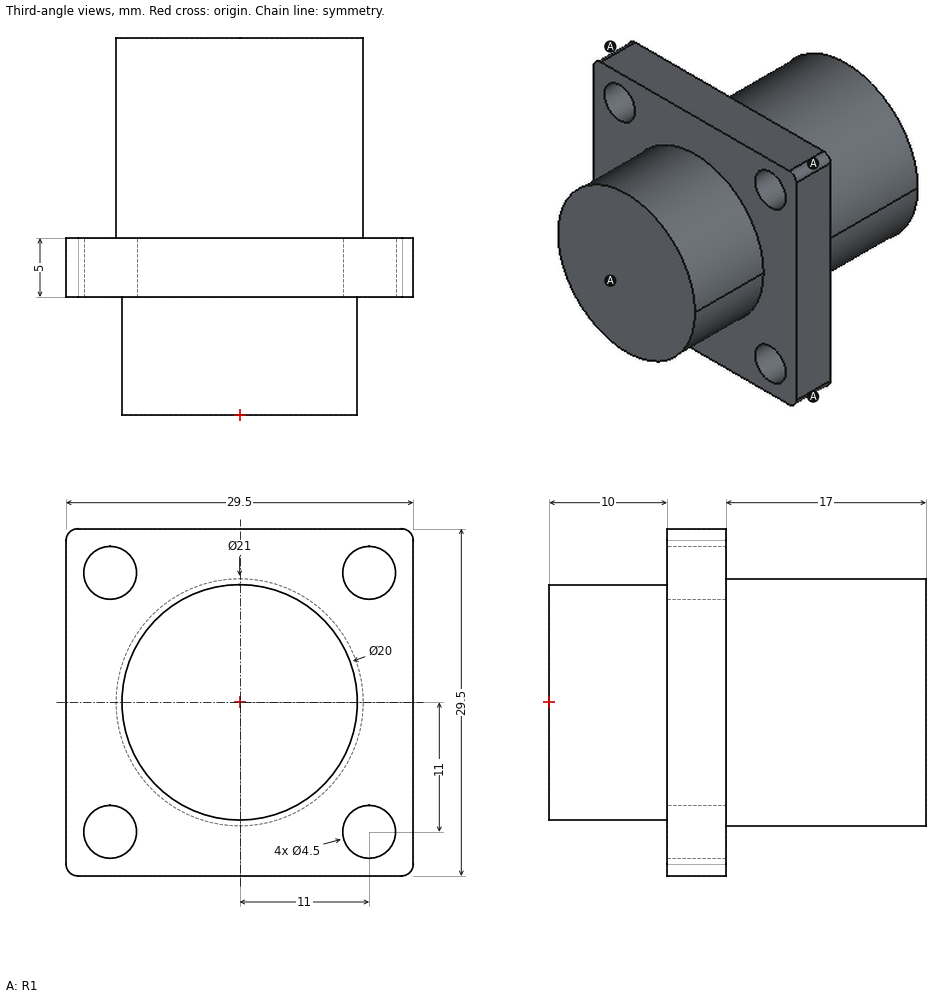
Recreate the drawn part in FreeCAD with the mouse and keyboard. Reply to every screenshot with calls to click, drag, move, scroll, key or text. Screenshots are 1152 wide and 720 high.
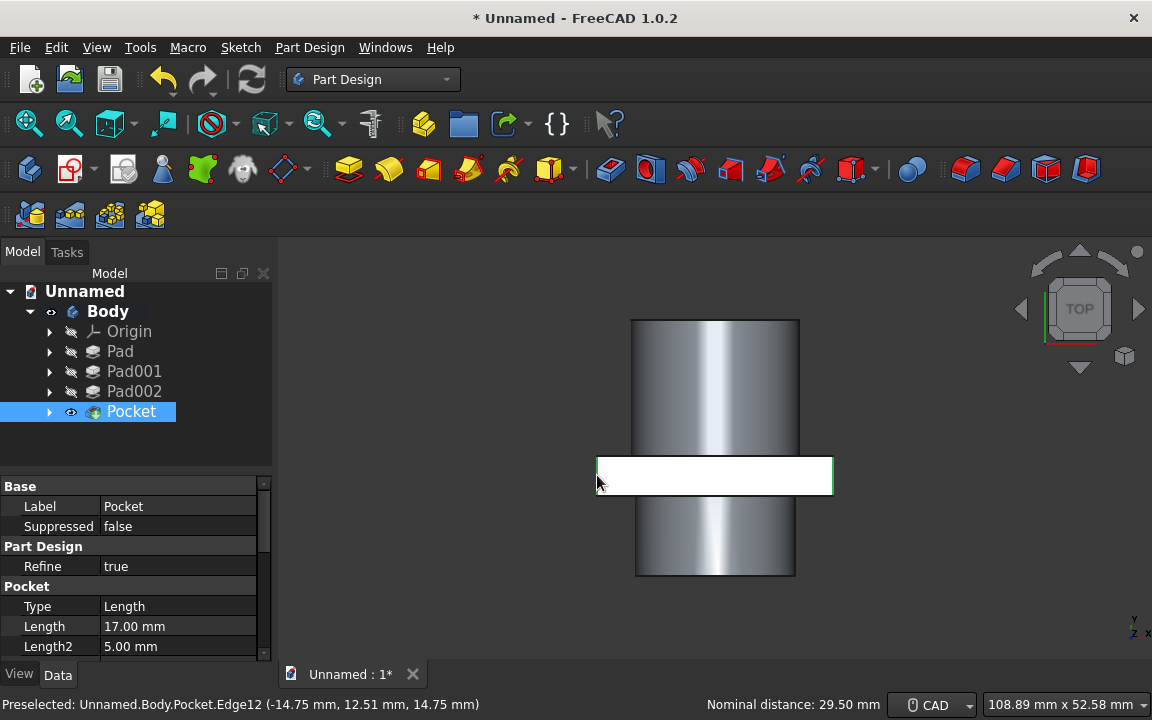
key(1)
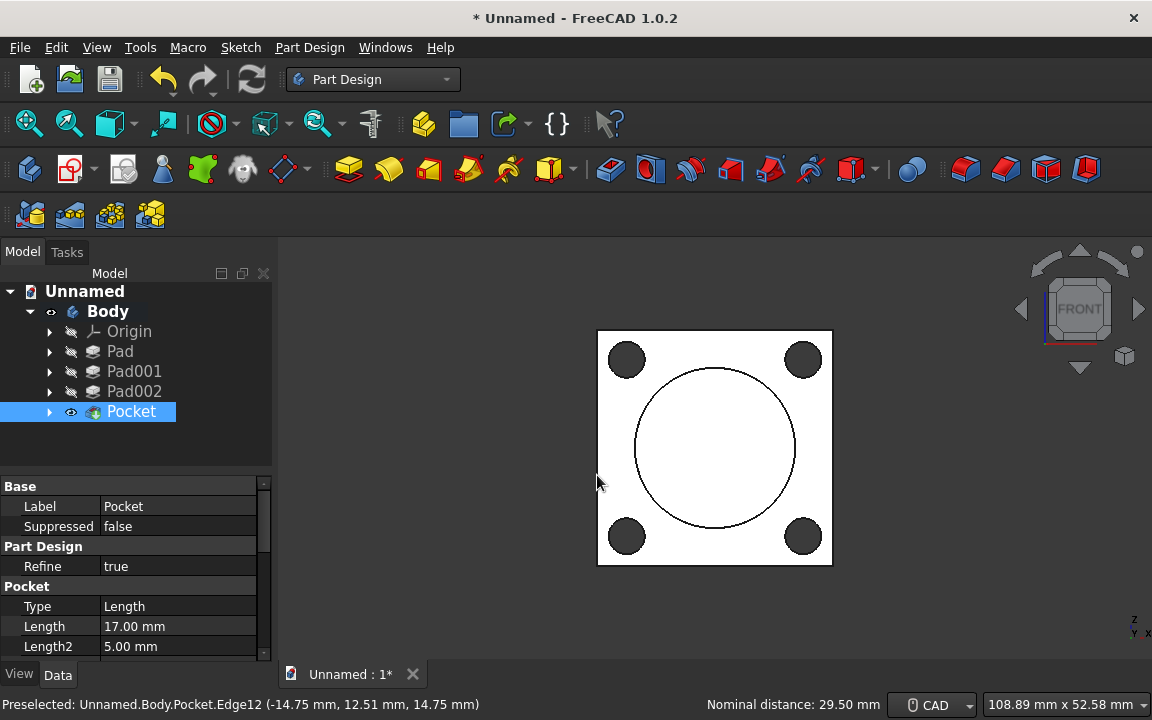
key(3)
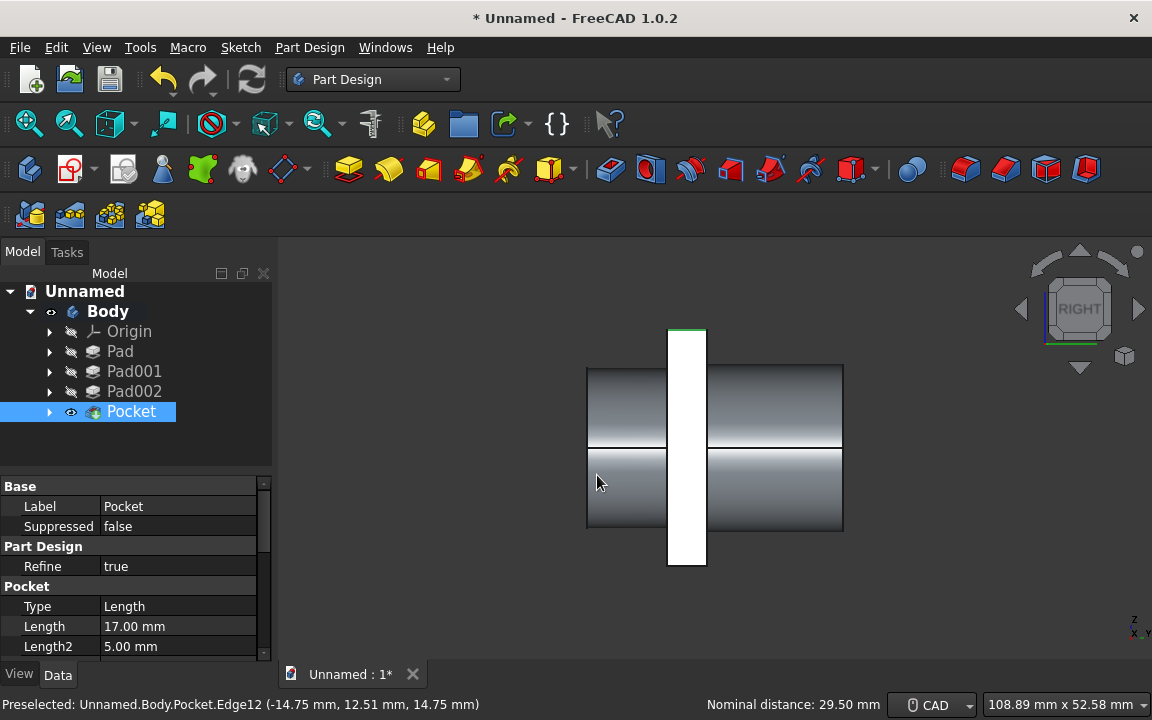
click(687, 565, ctrl)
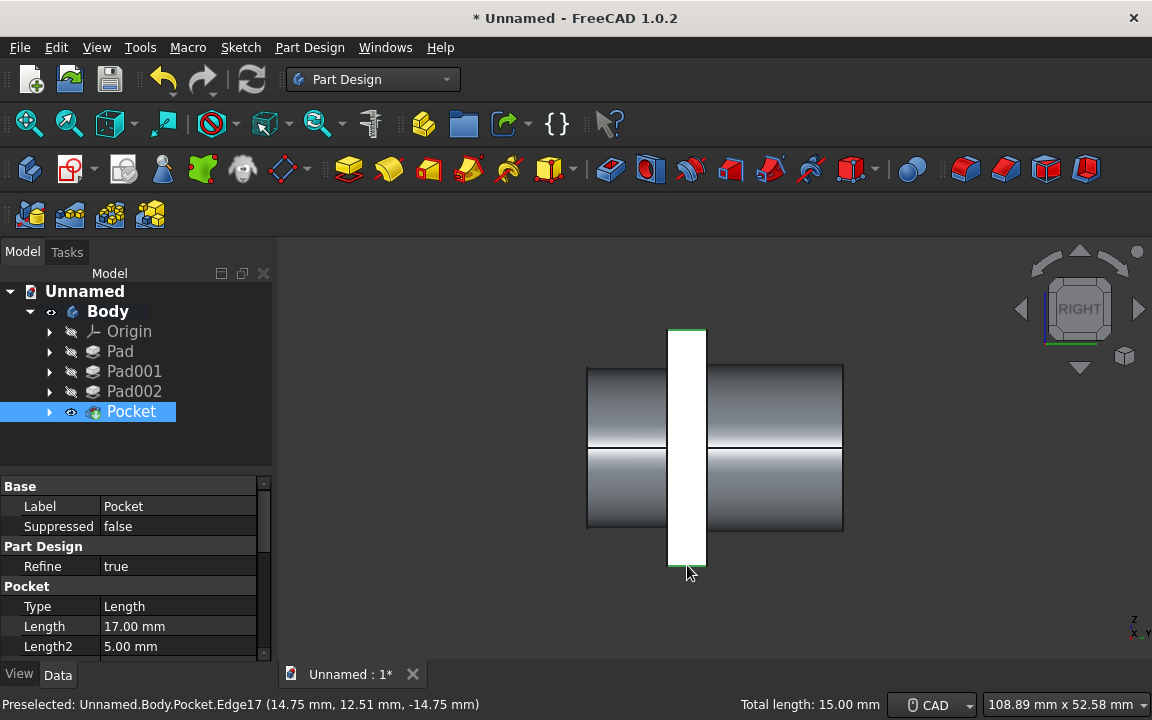
key(5)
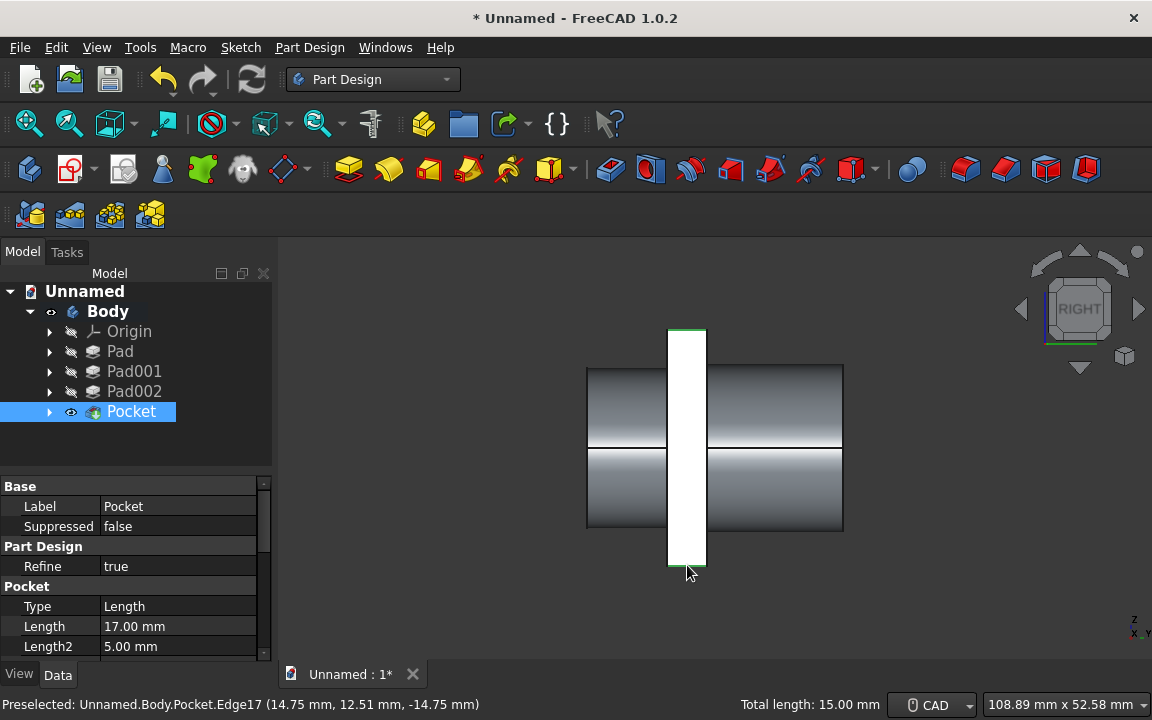
click(597, 419, ctrl)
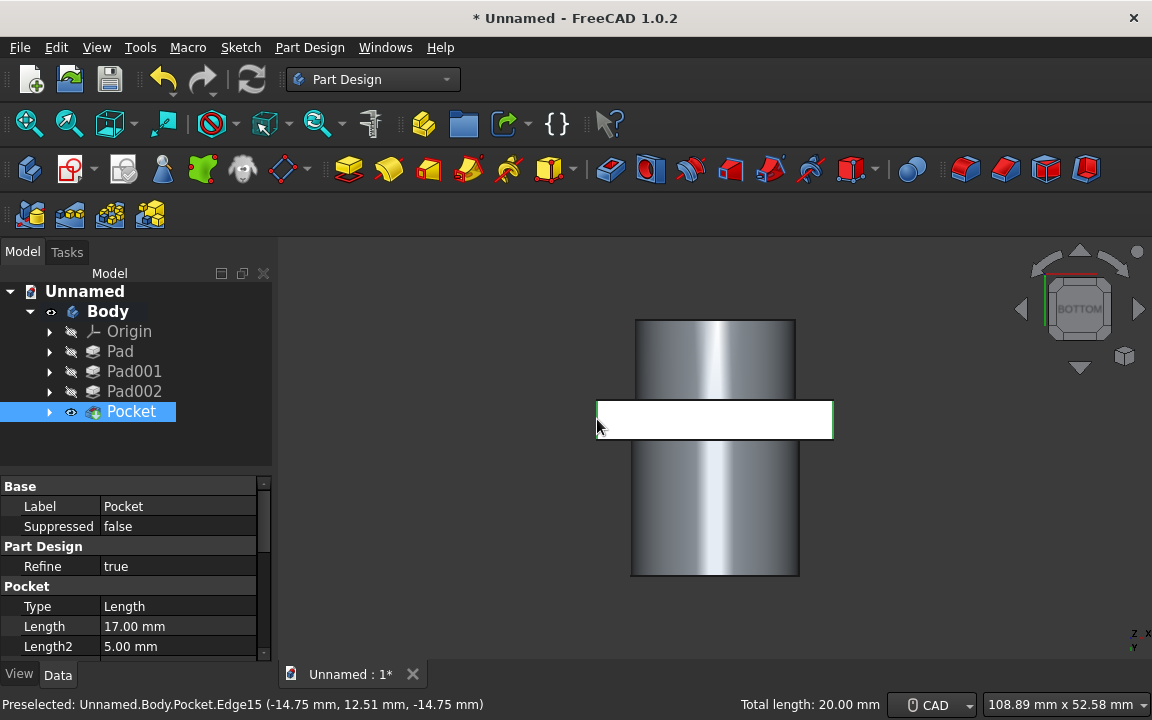
click(966, 170)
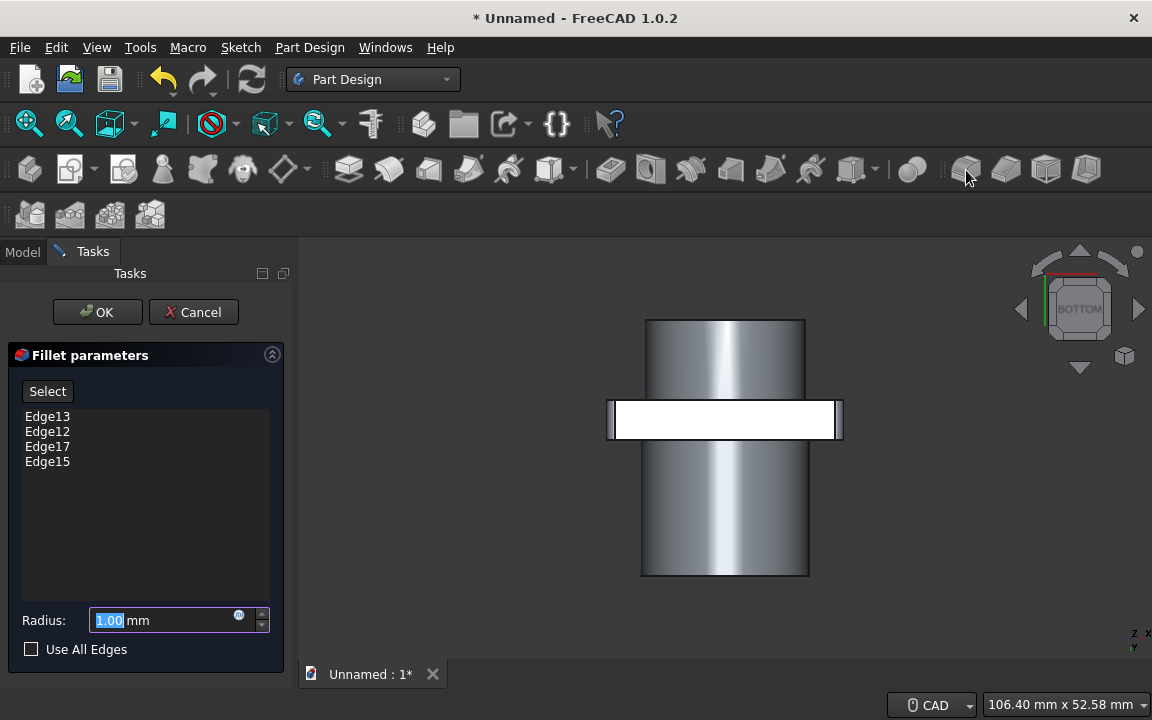
text(1)
key(Tab)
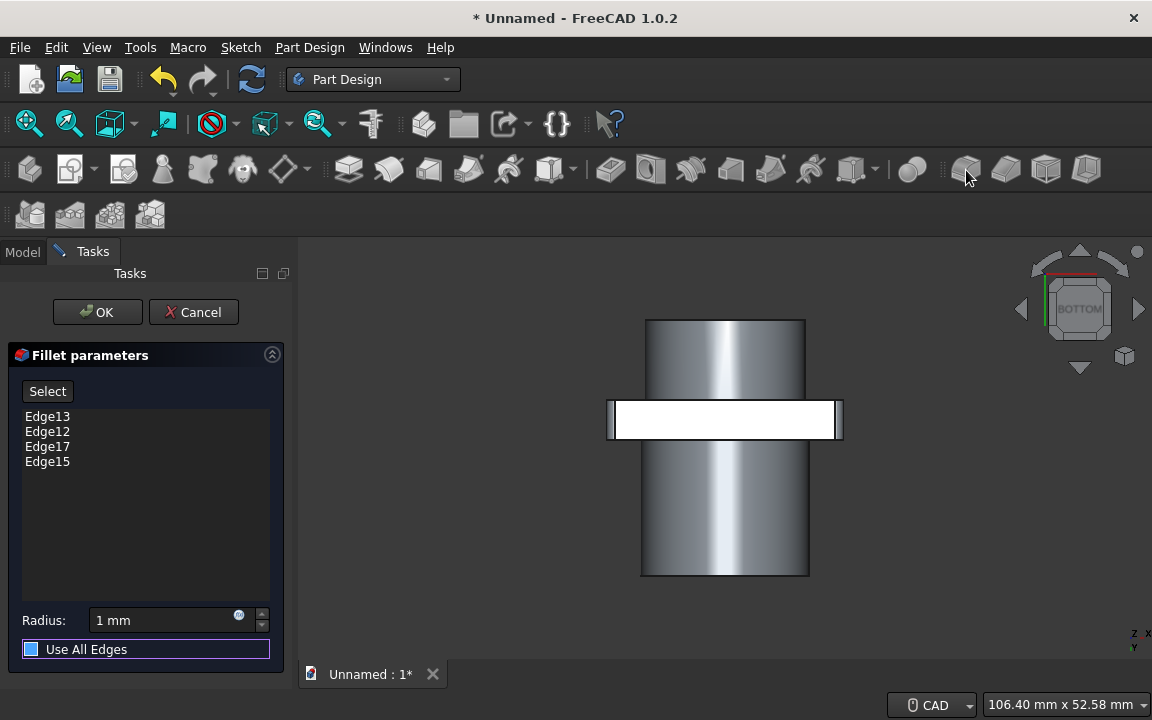
click(98, 312)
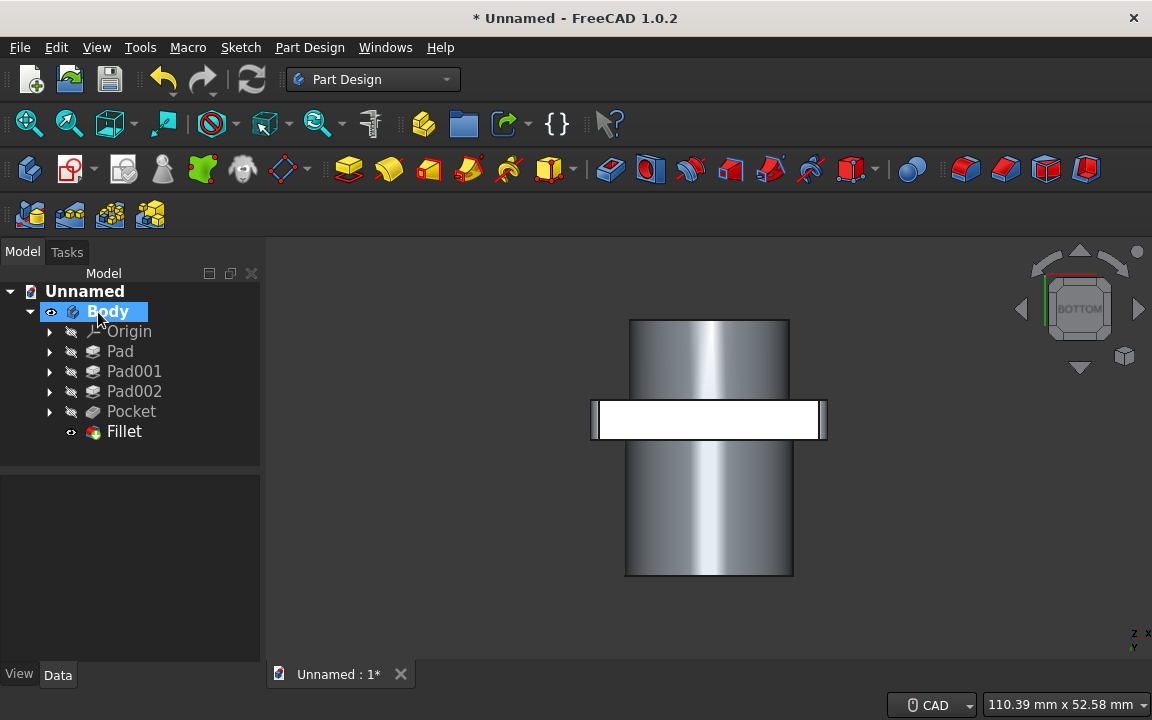
key(0)